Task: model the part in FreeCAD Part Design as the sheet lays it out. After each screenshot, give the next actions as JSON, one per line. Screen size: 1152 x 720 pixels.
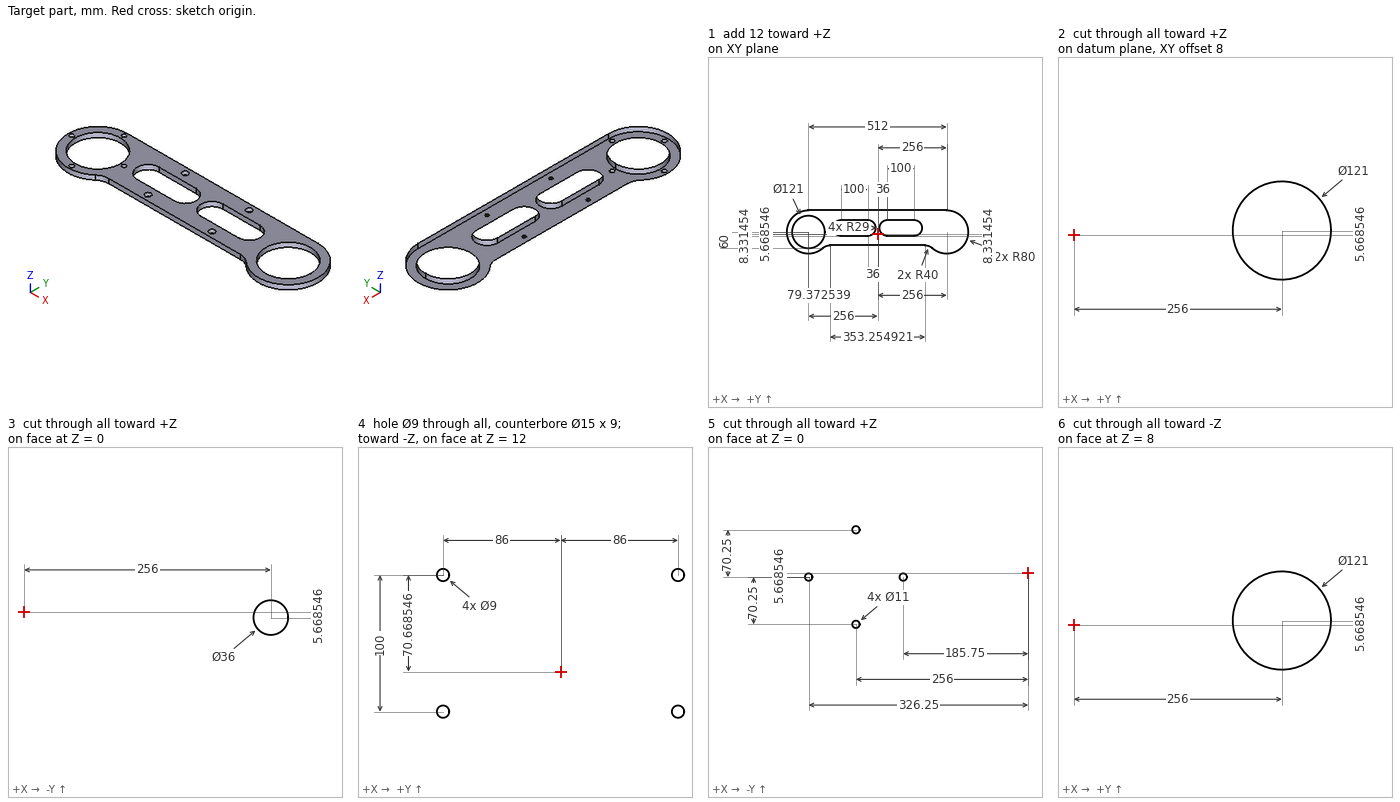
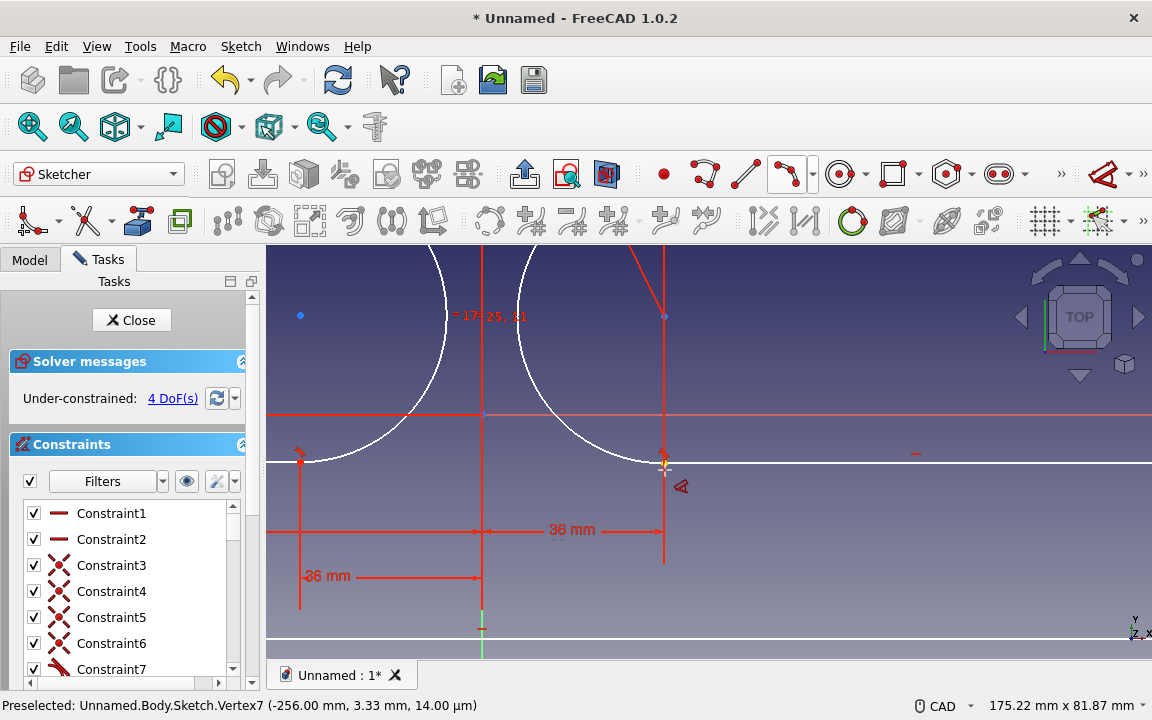
{"action": "left_click", "coordinate": [664, 463]}
{"action": "left_click", "coordinate": [698, 439]}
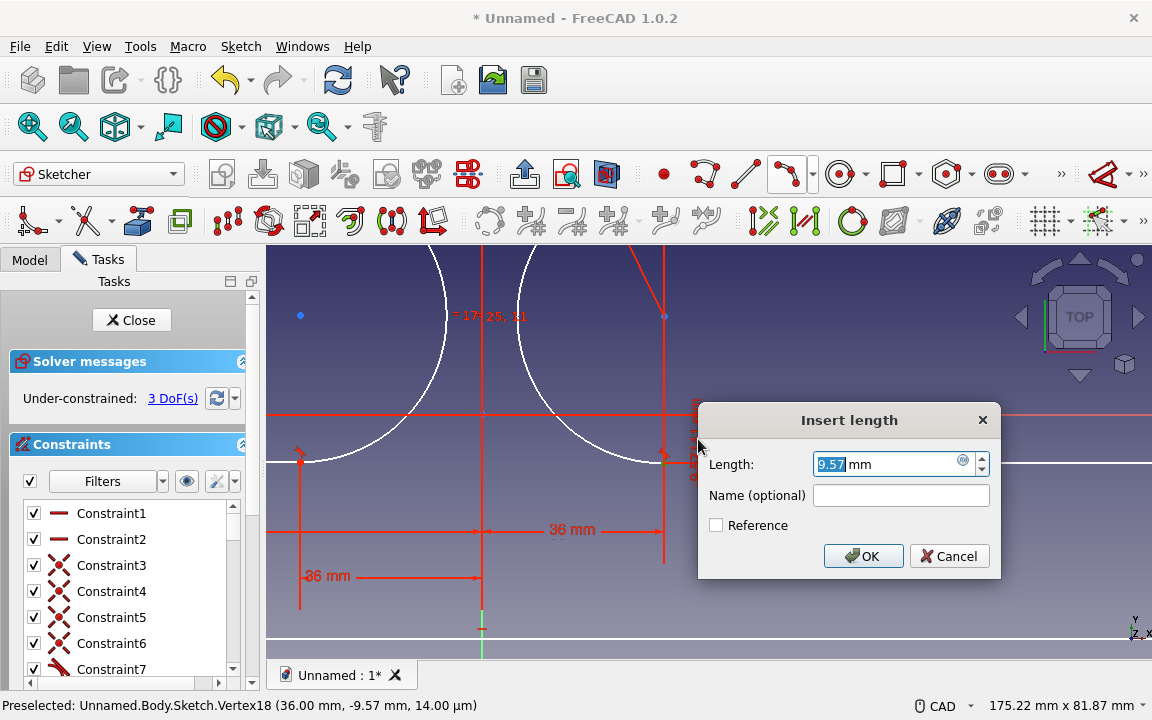
{"action": "type", "text": "8.331454"}
{"action": "key", "text": "Return"}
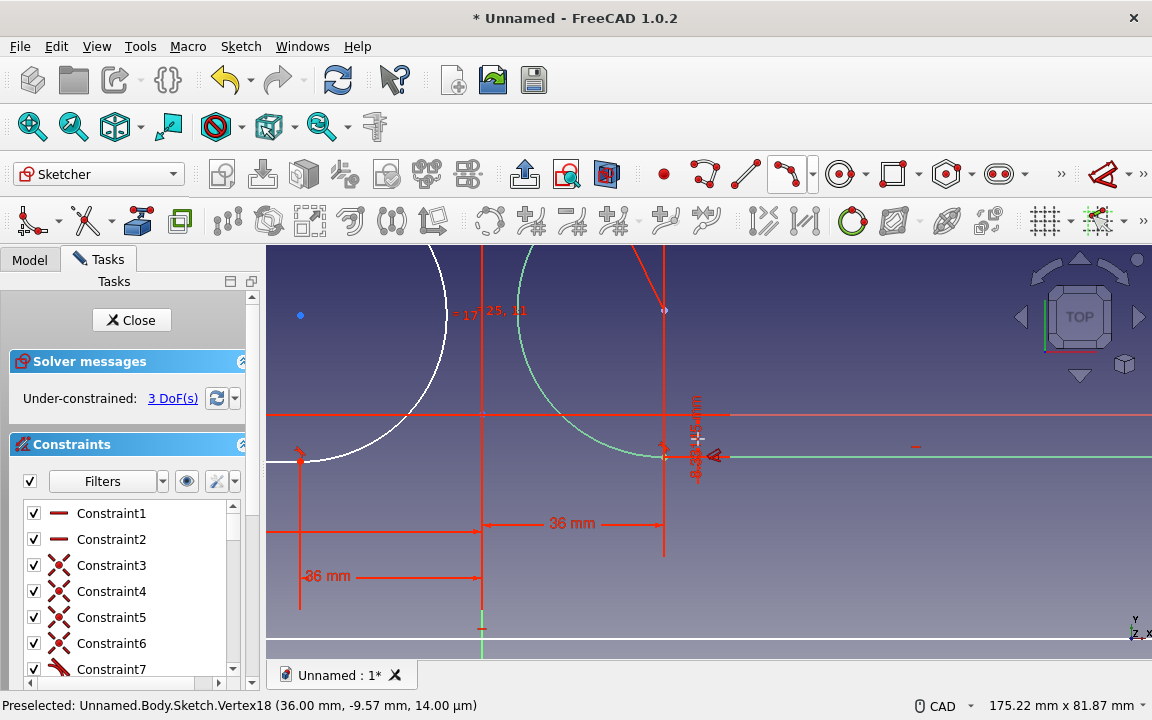
{"action": "scroll", "coordinate": [665, 470], "scroll_direction": "down", "scroll_amount": 10}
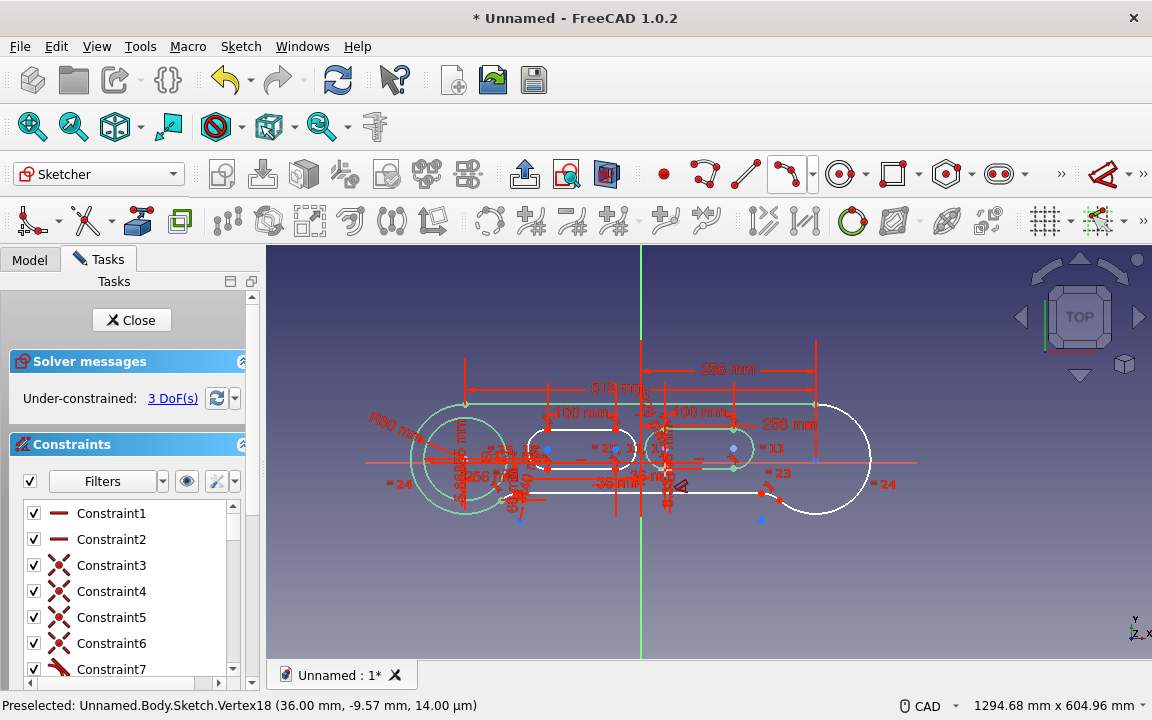
{"action": "scroll", "coordinate": [548, 469], "scroll_direction": "up", "scroll_amount": 10}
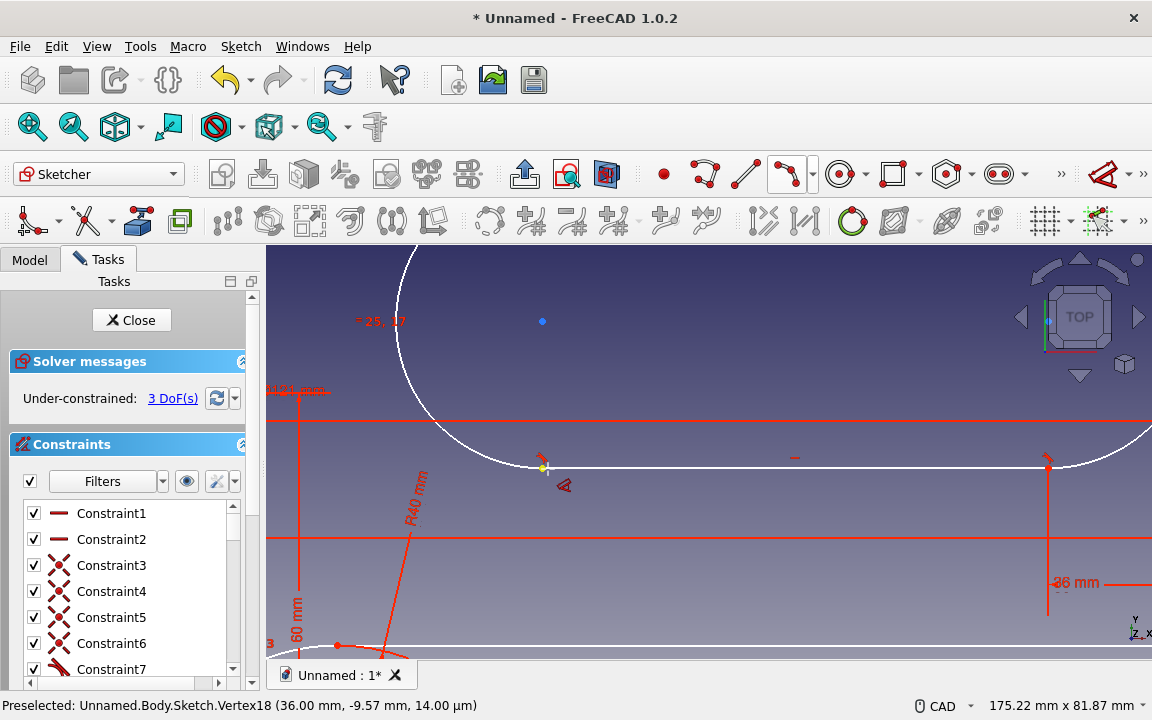
{"action": "left_click", "coordinate": [543, 468]}
{"action": "left_click", "coordinate": [509, 445]}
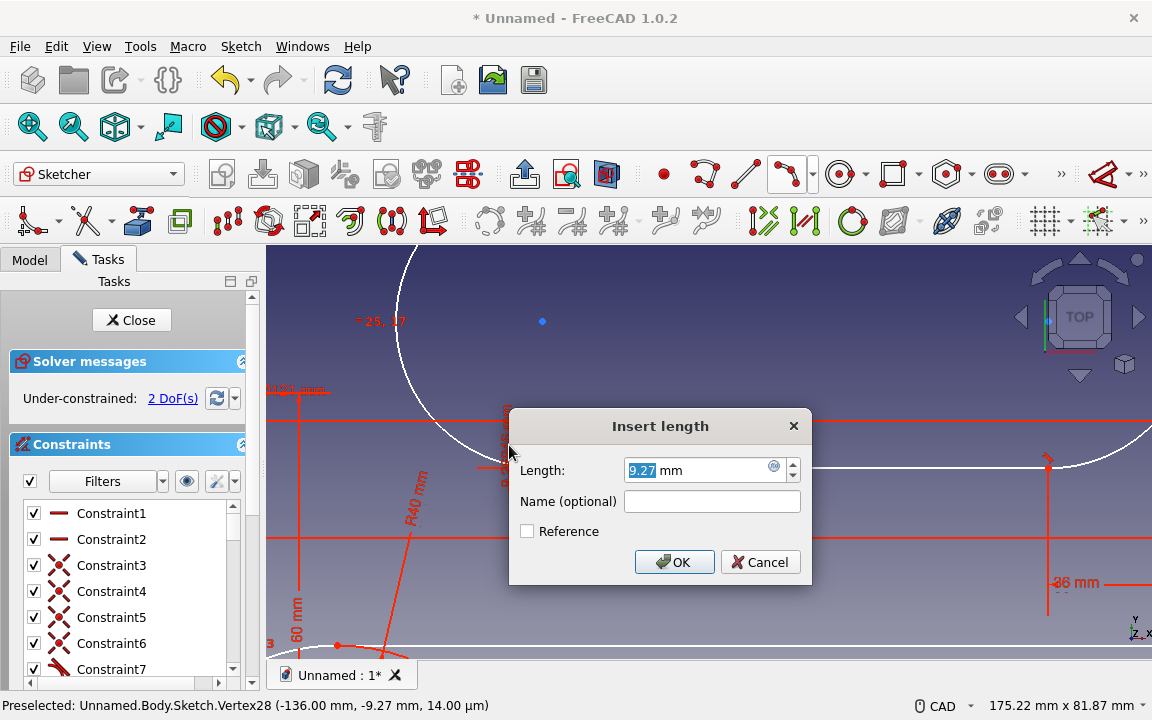
{"action": "type", "text": "8.331454"}
{"action": "key", "text": "Return"}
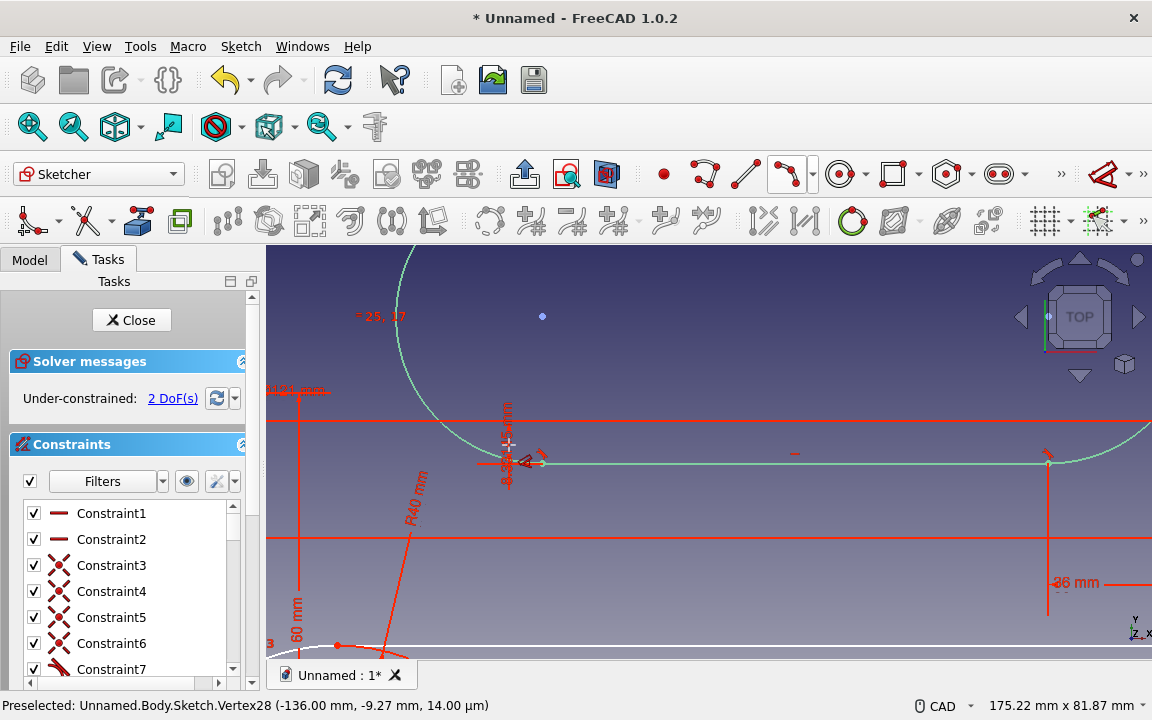
{"action": "scroll", "coordinate": [548, 469], "scroll_direction": "down", "scroll_amount": 10}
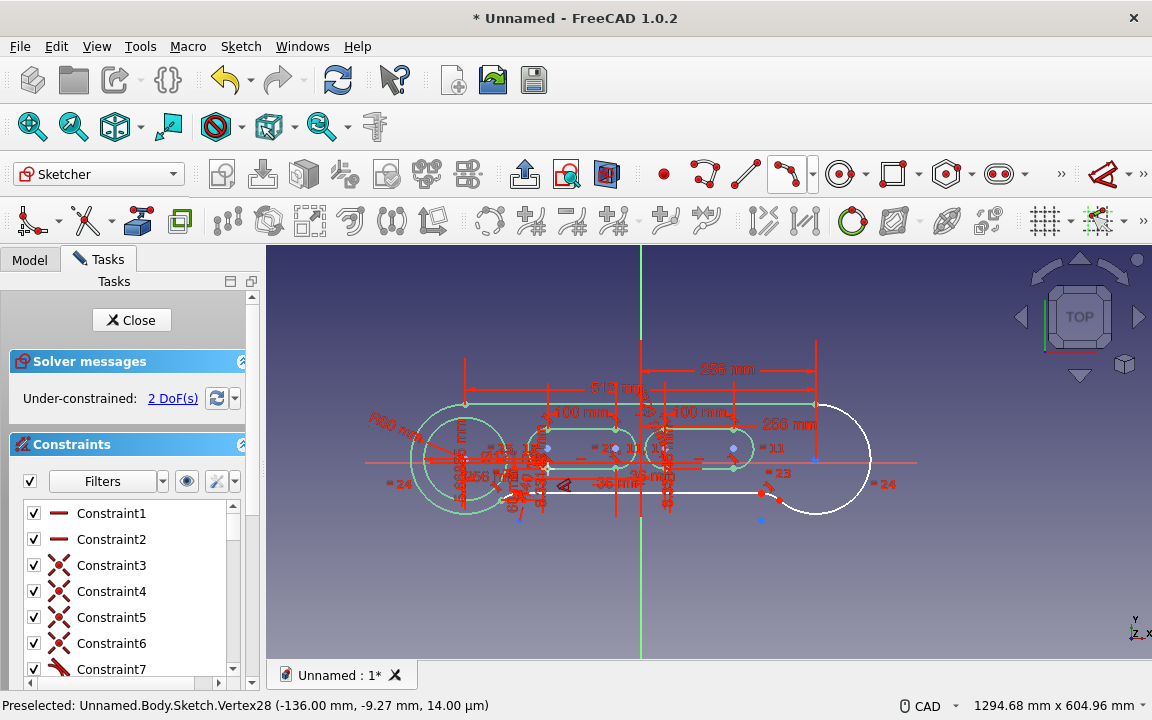
{"action": "left_click", "coordinate": [592, 493]}
{"action": "left_click", "coordinate": [585, 527]}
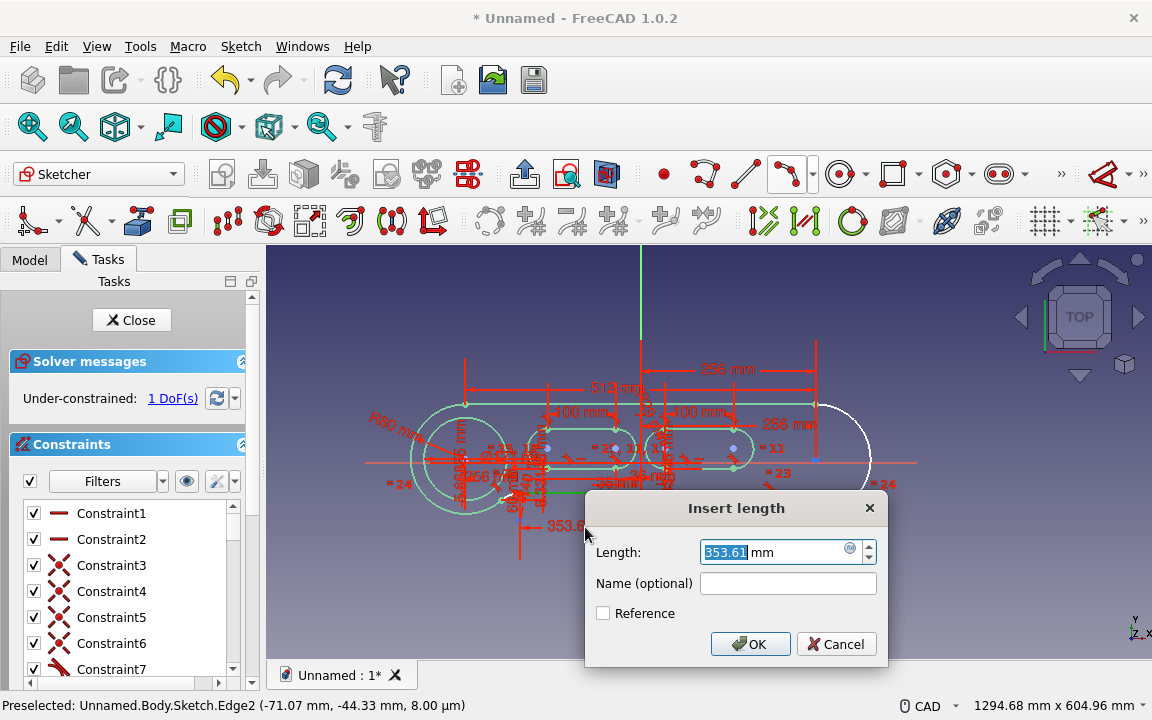
{"action": "type", "text": "353.254921"}
{"action": "key", "text": "Return"}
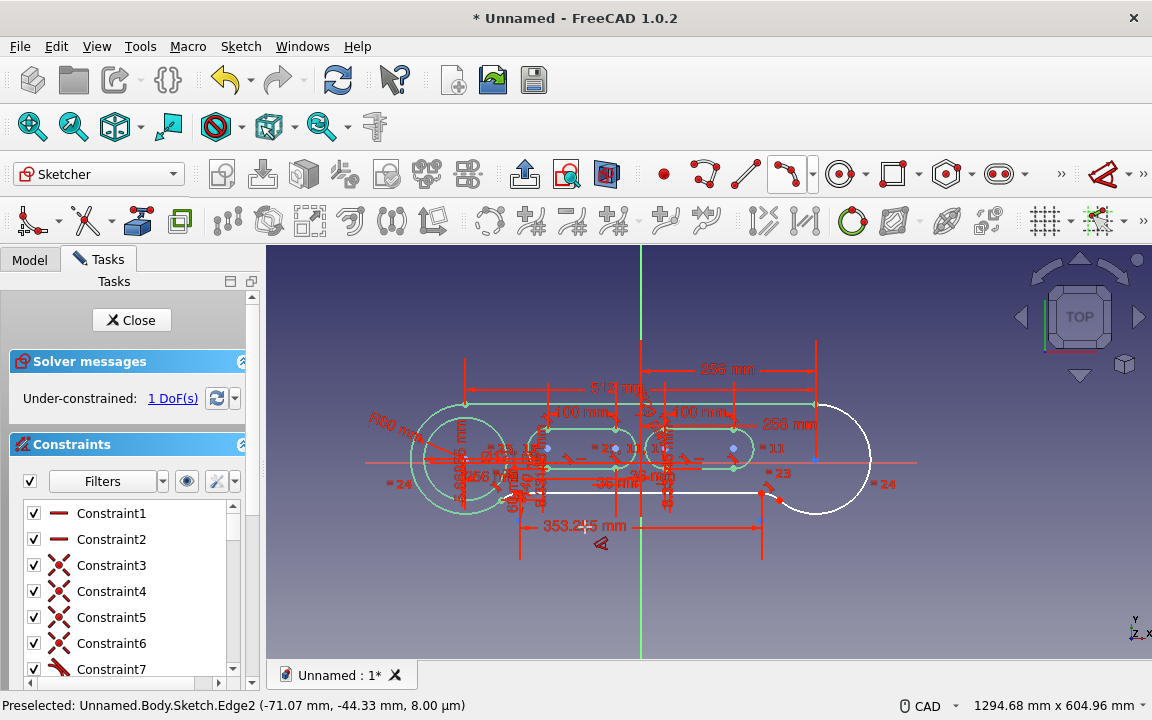
{"action": "left_click", "coordinate": [520, 493]}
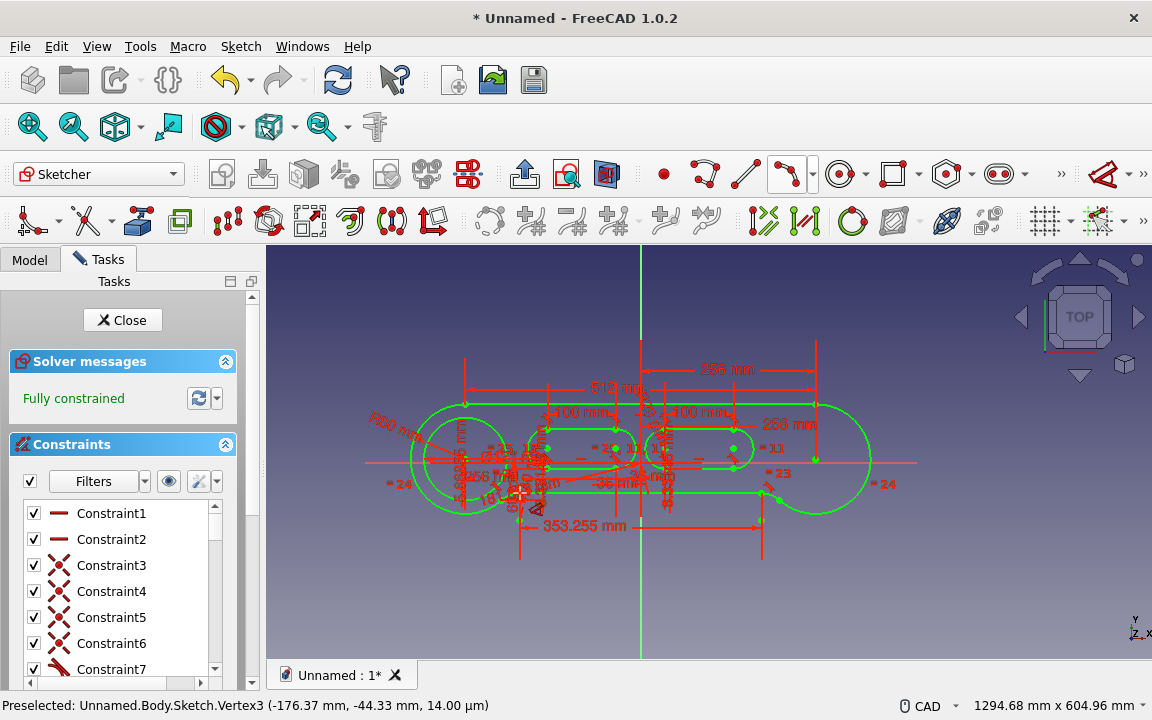
{"action": "left_click", "coordinate": [465, 459]}
{"action": "left_click", "coordinate": [493, 527]}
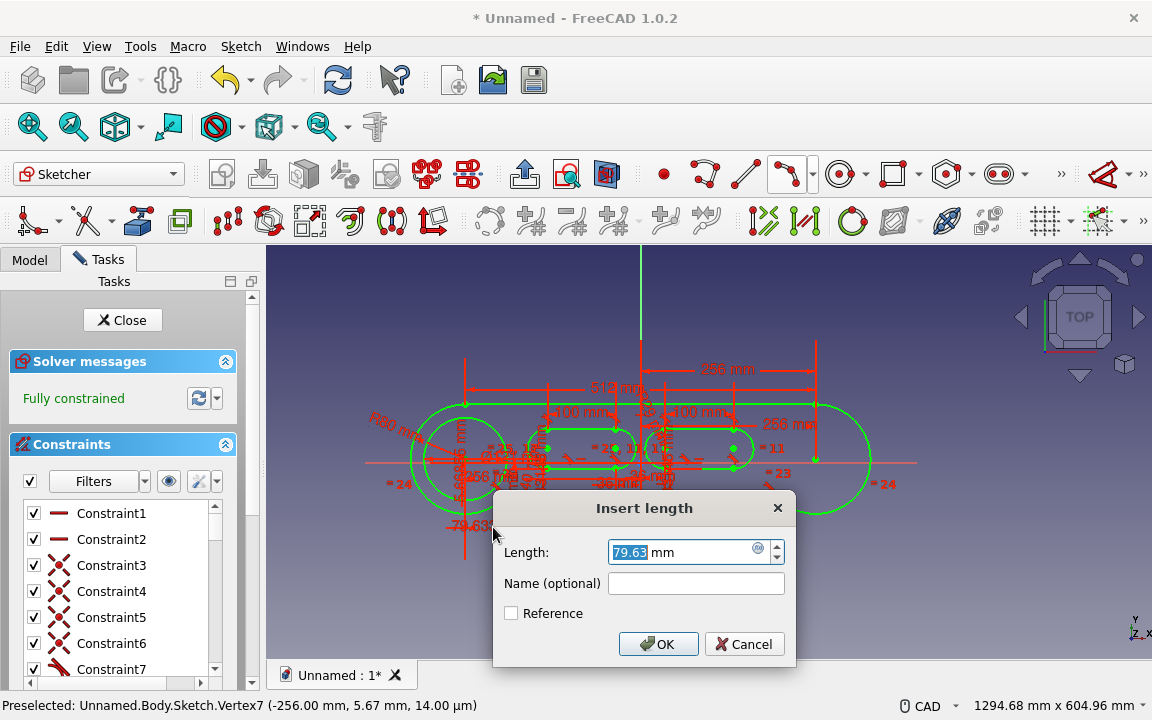
{"action": "type", "text": "79.372539"}
{"action": "key", "text": "Return"}
{"action": "key", "text": "Escape"}